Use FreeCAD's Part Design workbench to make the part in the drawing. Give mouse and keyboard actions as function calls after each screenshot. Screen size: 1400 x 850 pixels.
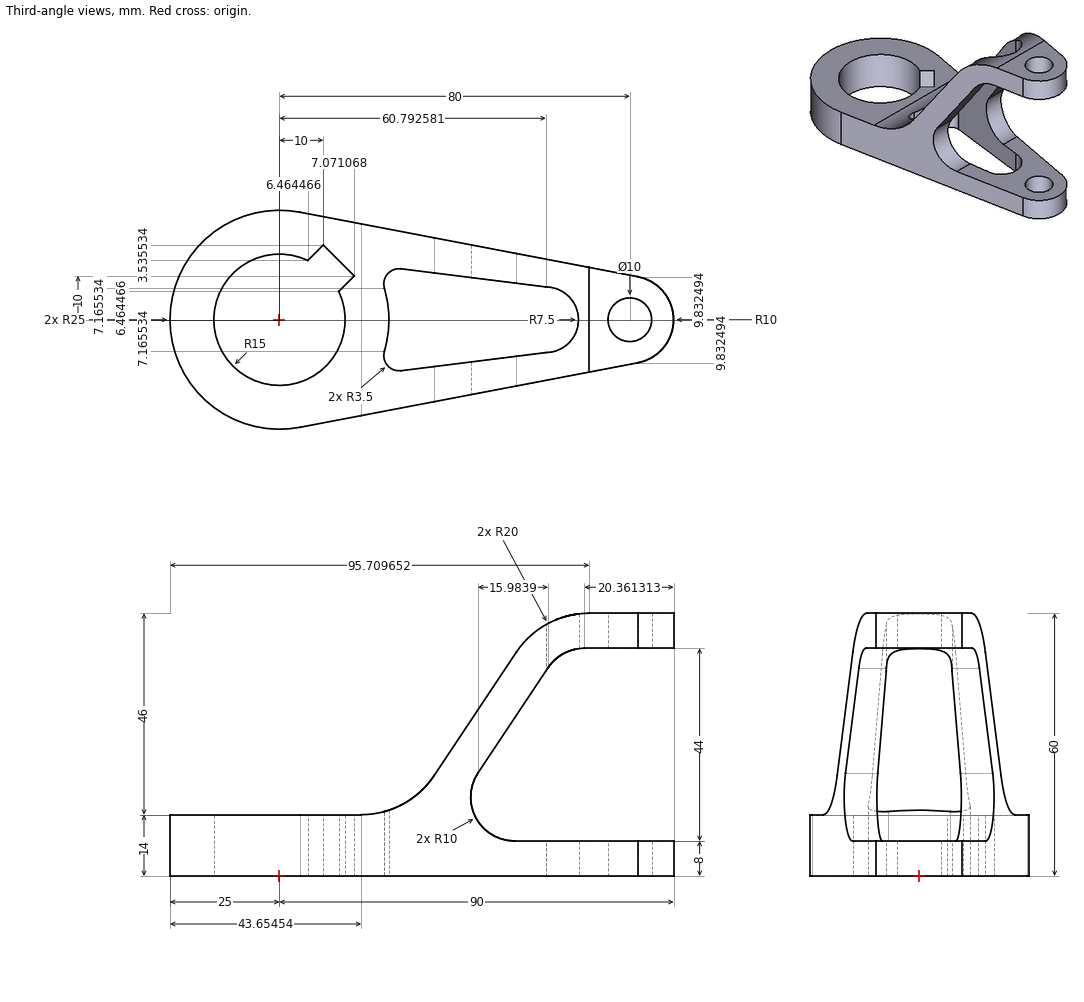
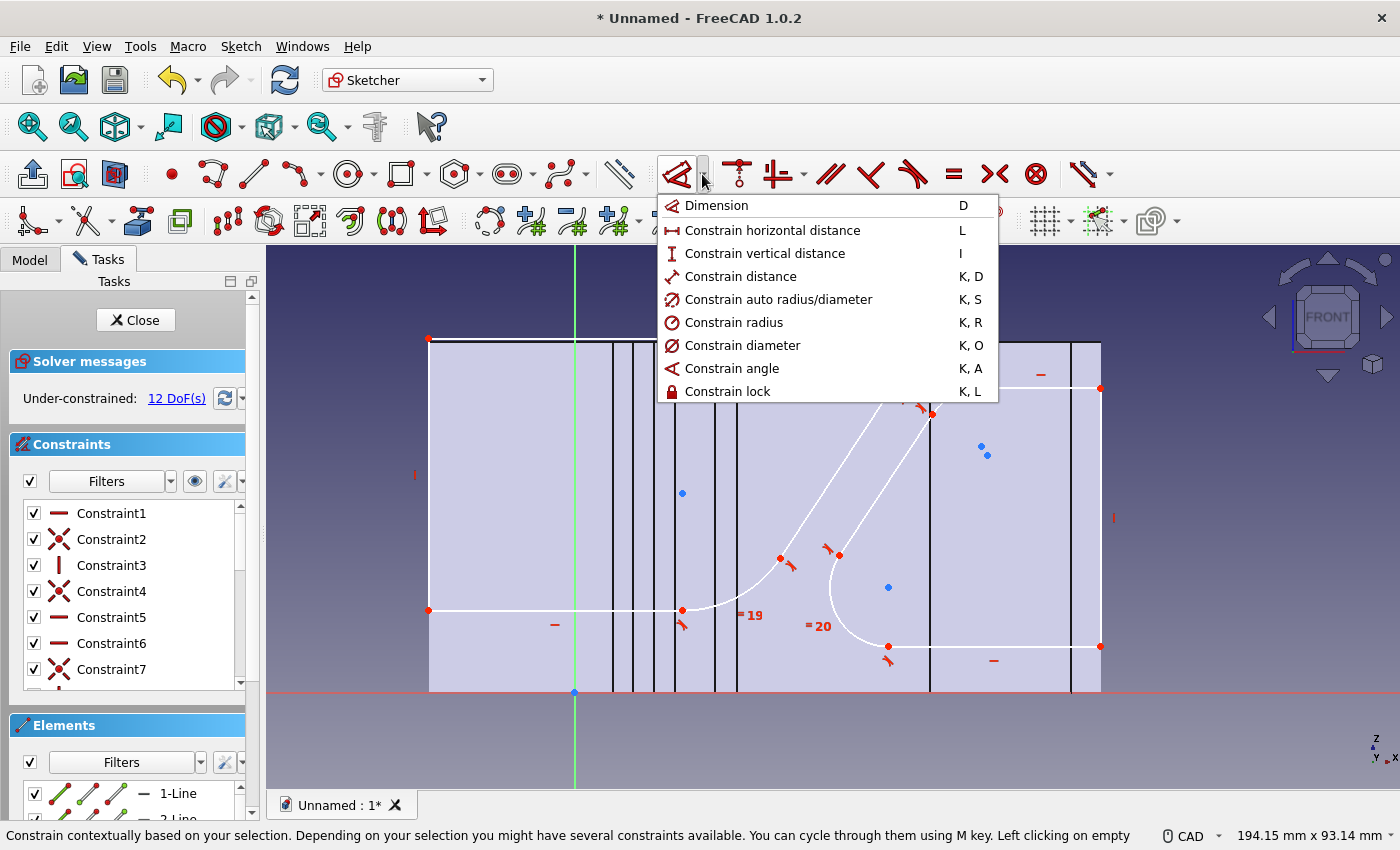
click(828, 322)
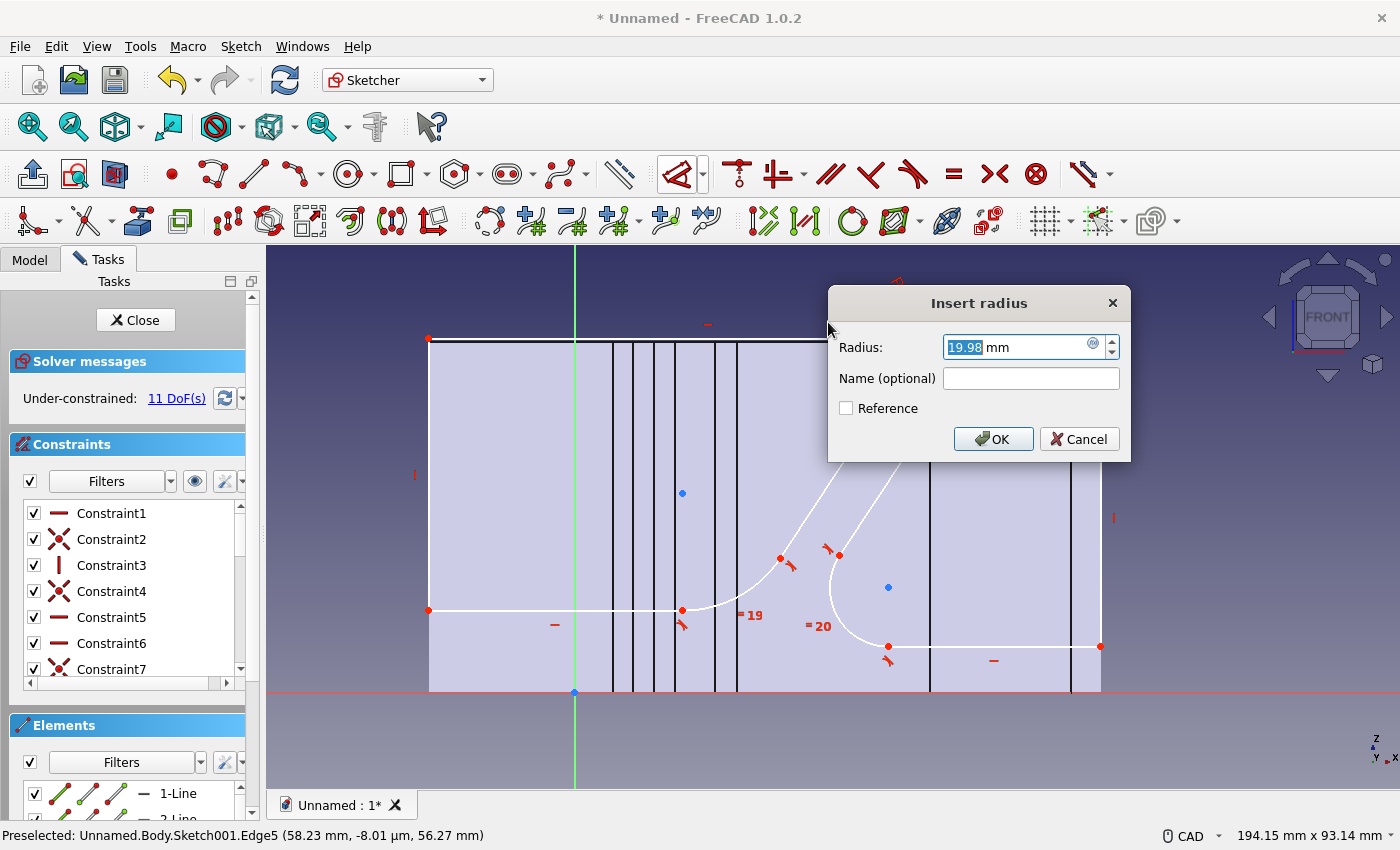
text(20)
key(Return)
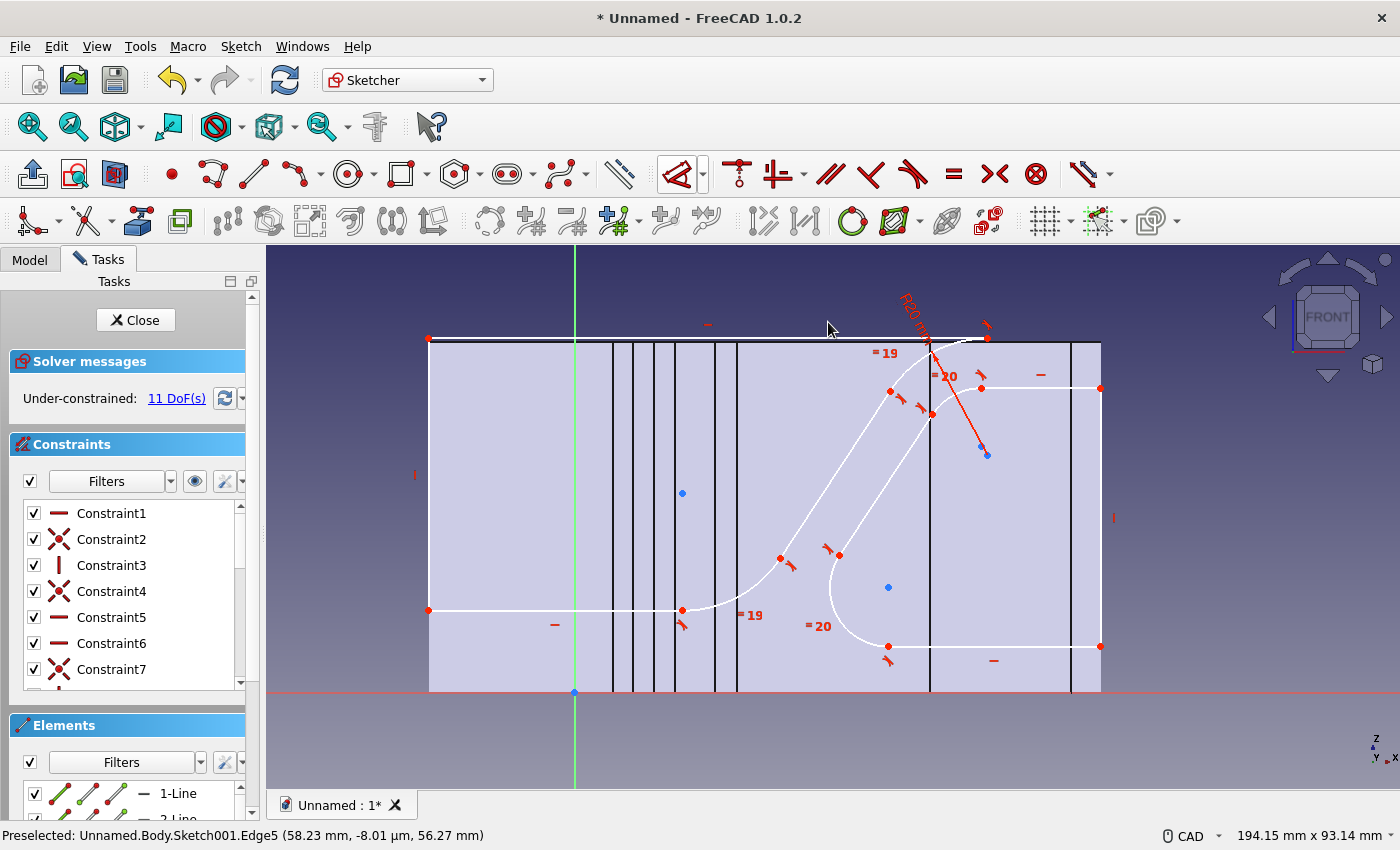
click(964, 391)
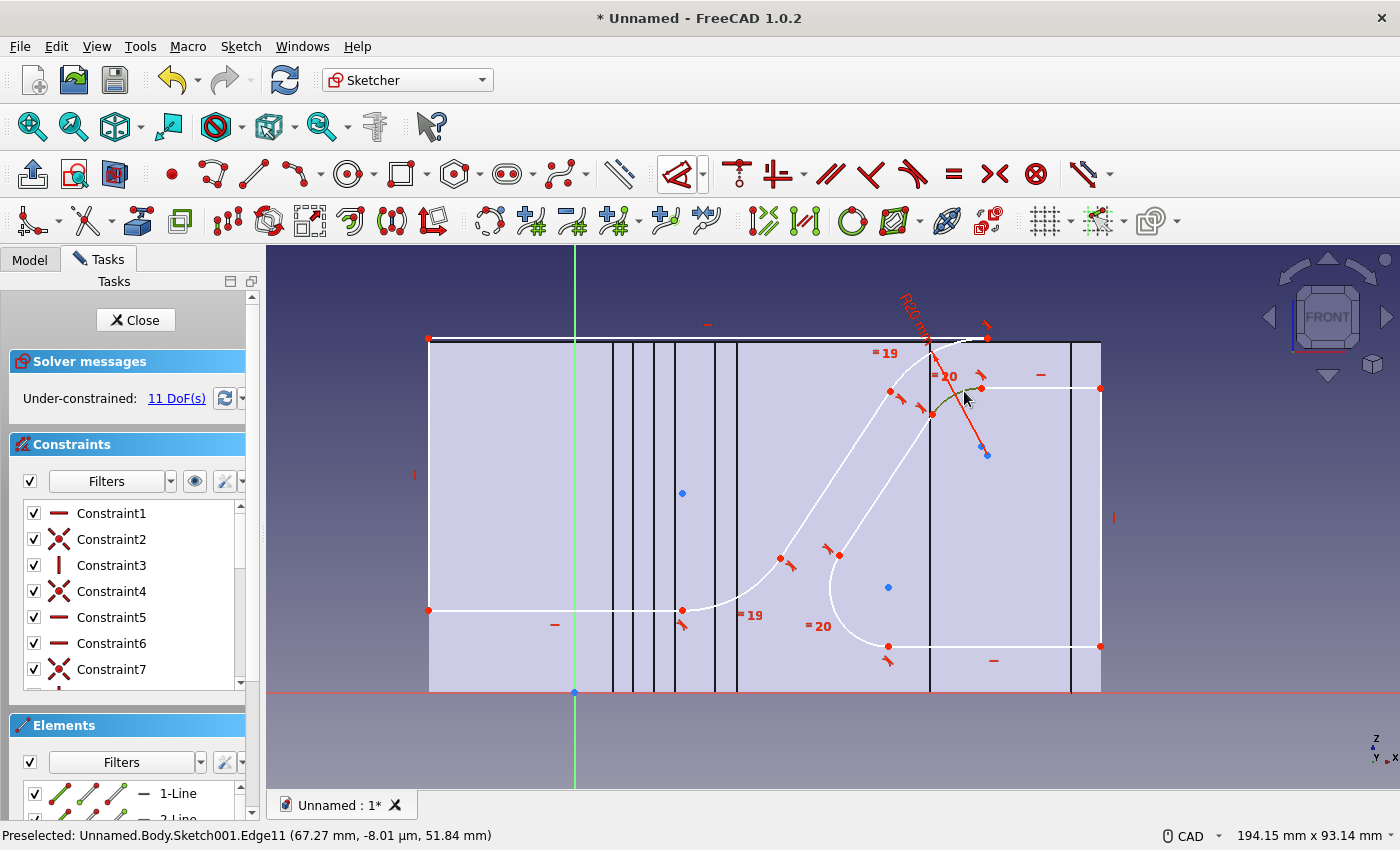
click(702, 174)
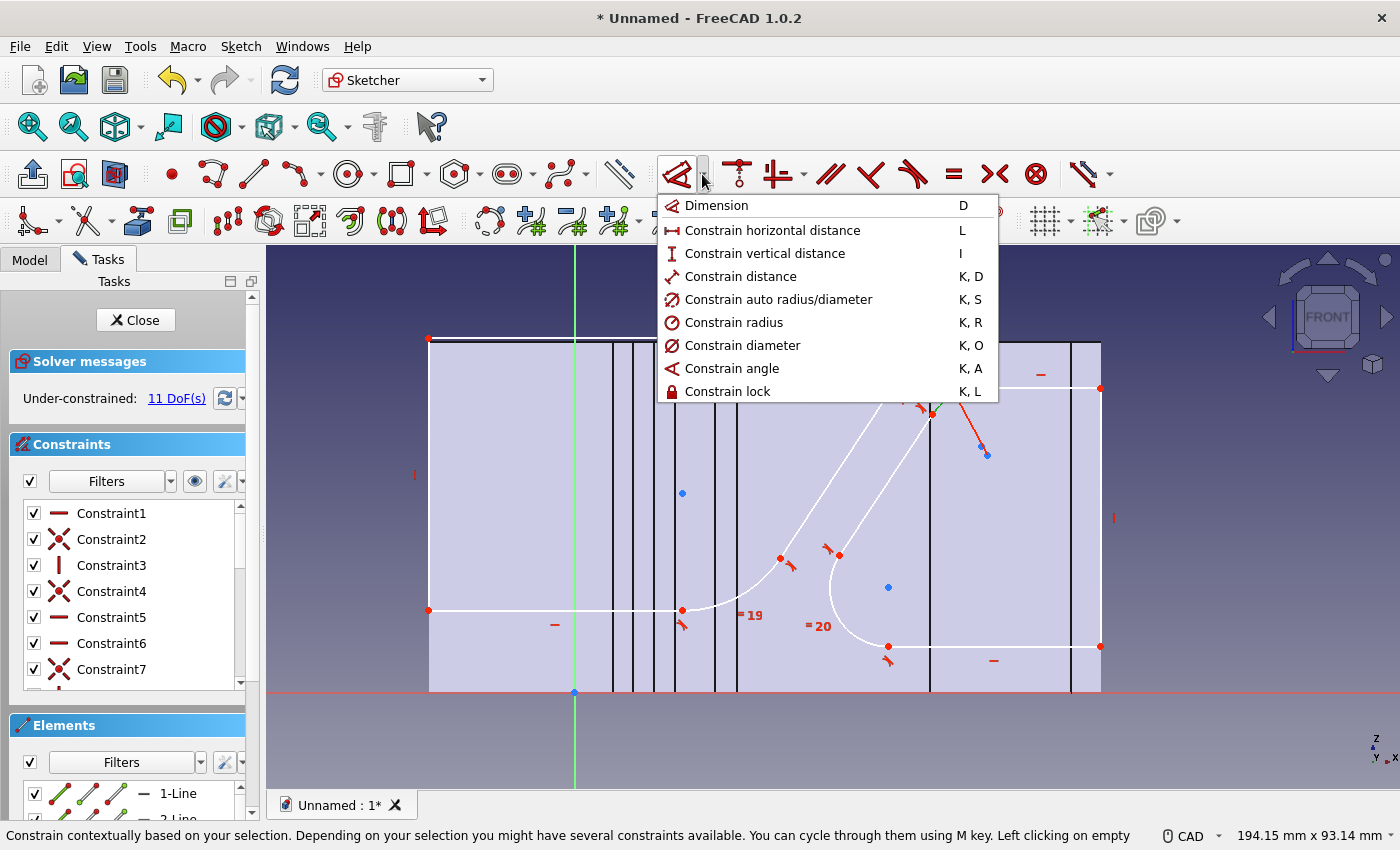
click(828, 322)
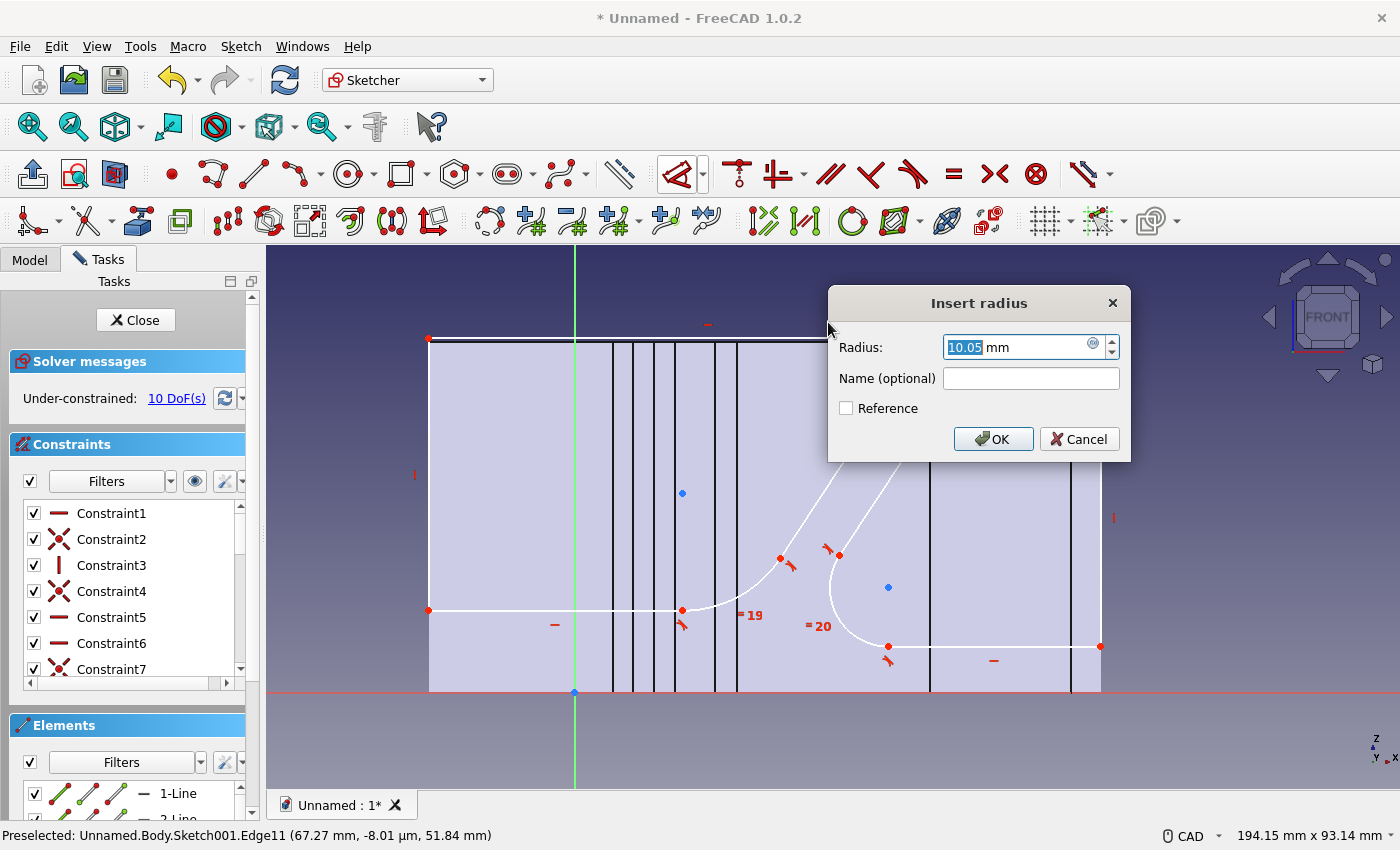
text(10)
key(Return)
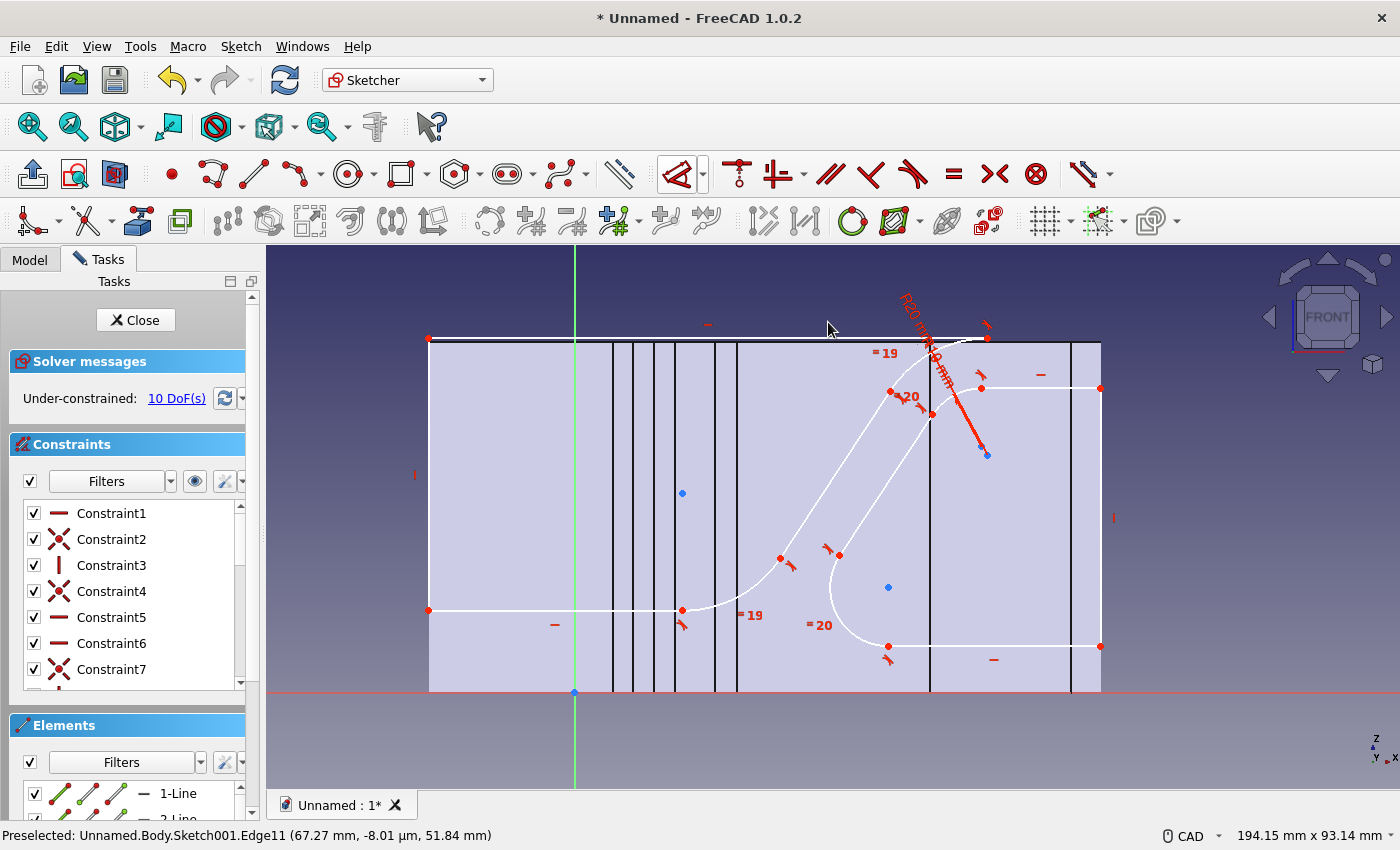
click(429, 529)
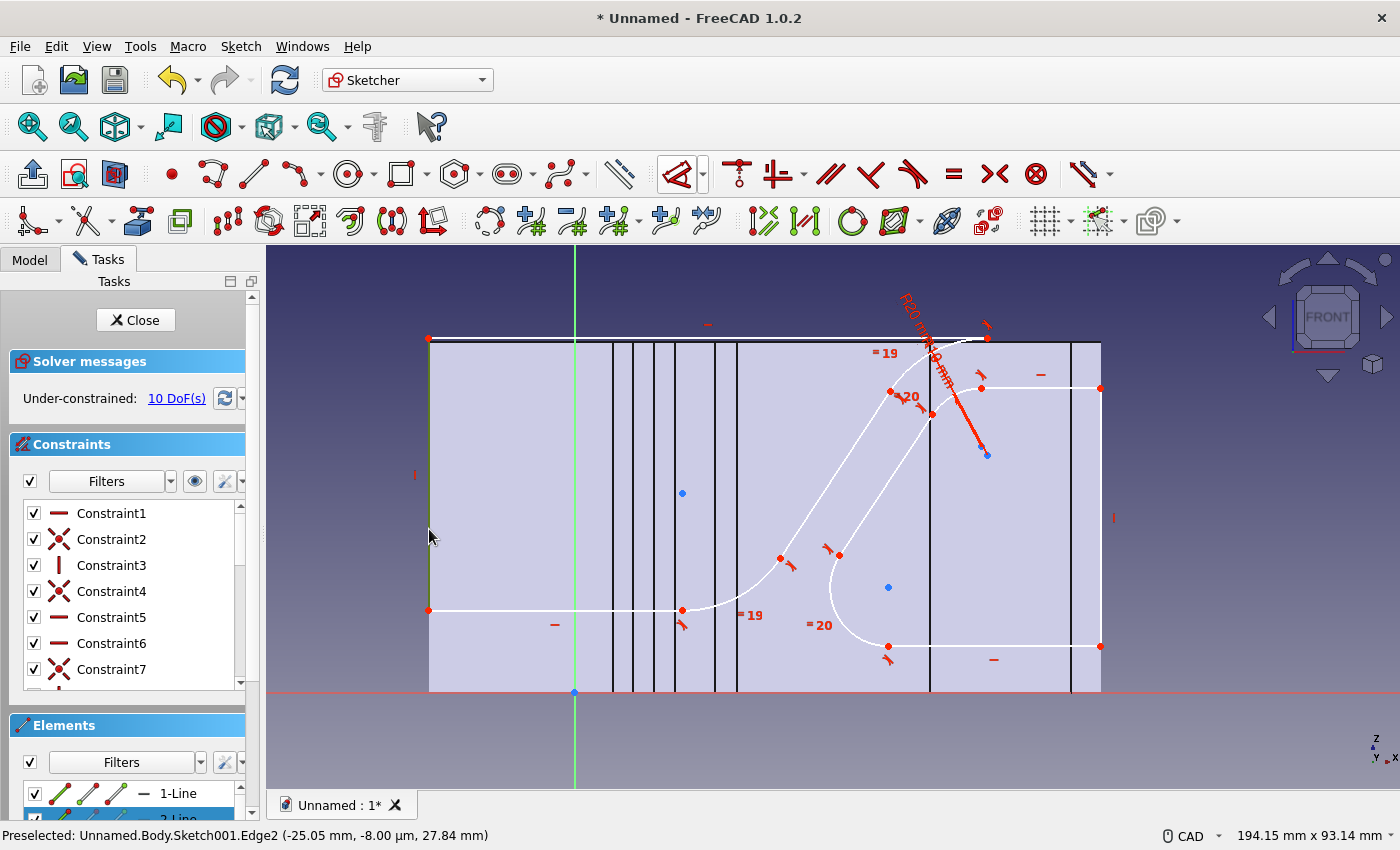
key(i)